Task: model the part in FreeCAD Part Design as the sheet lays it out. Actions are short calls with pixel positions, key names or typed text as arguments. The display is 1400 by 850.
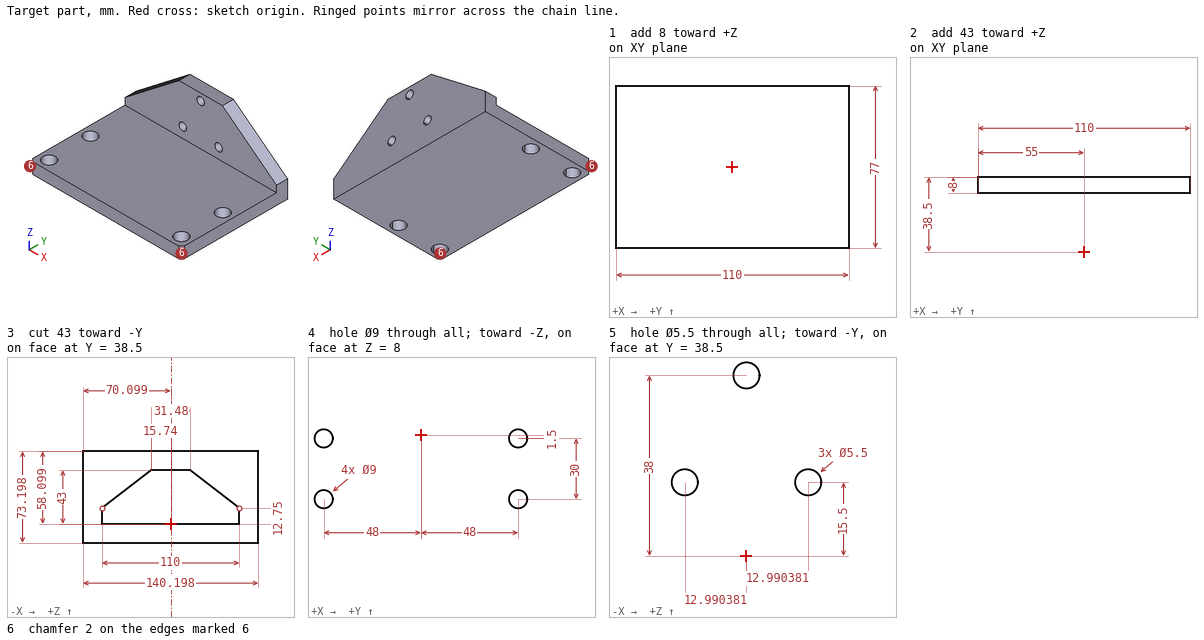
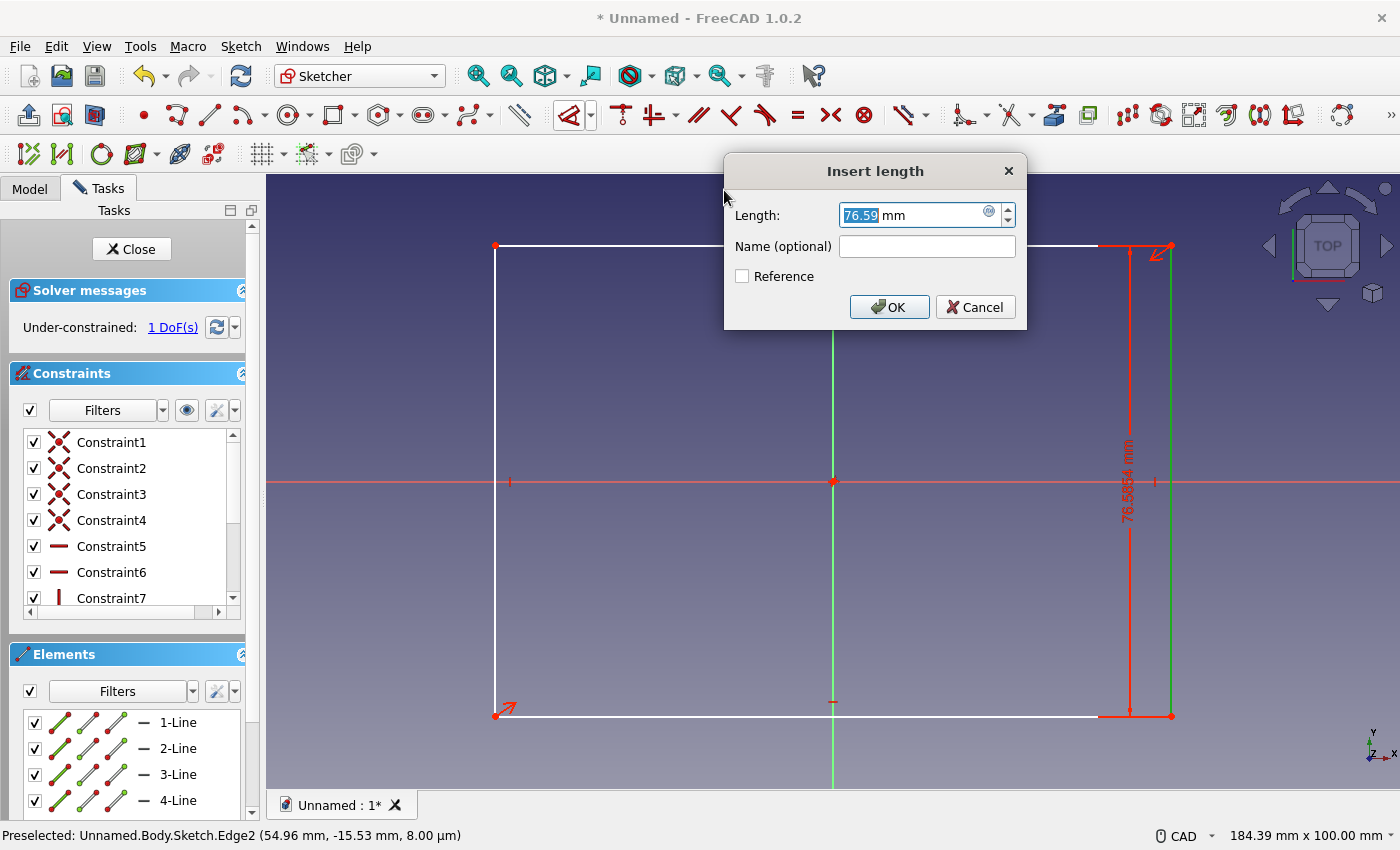
text(77)
key(Return)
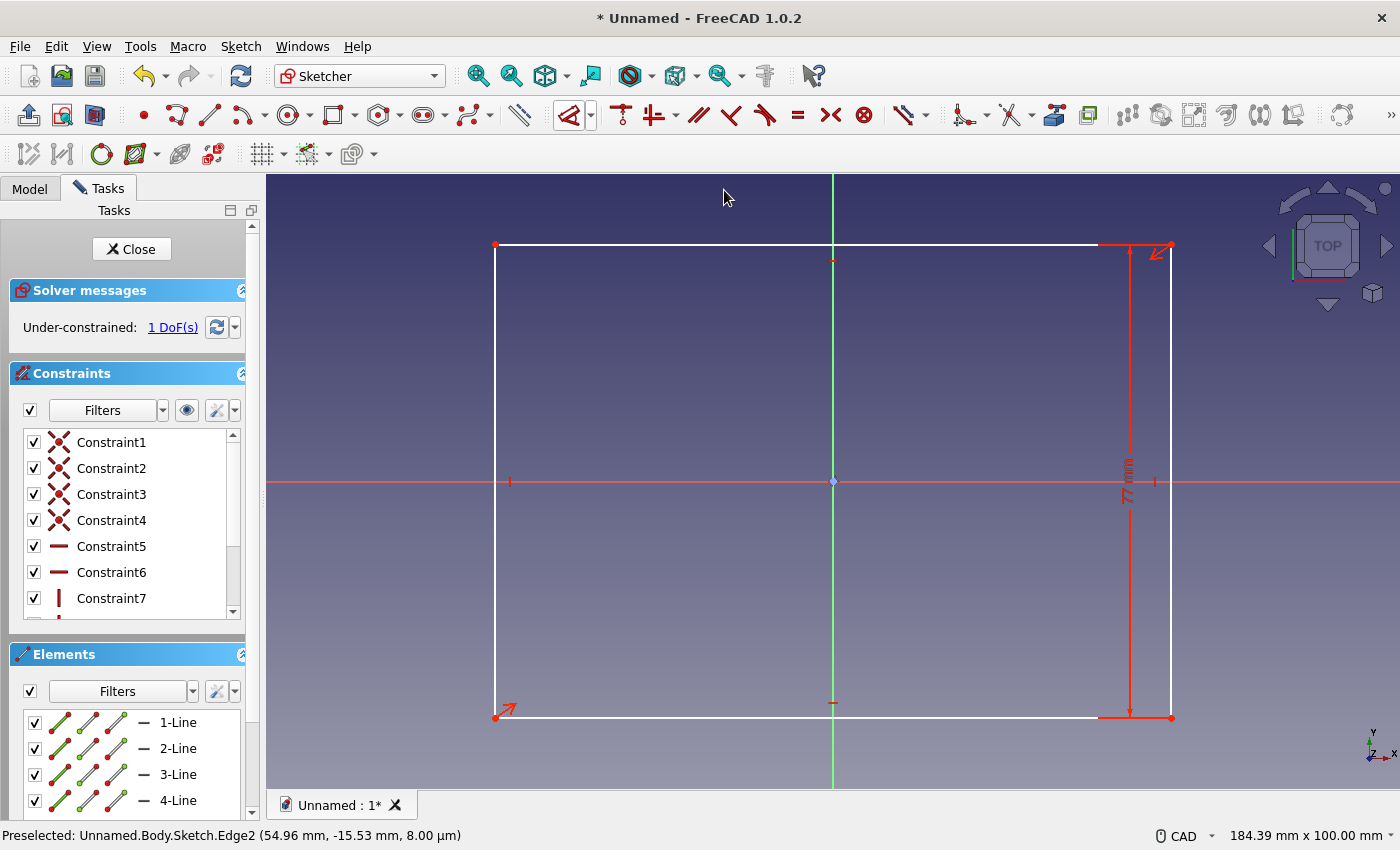
click(698, 718)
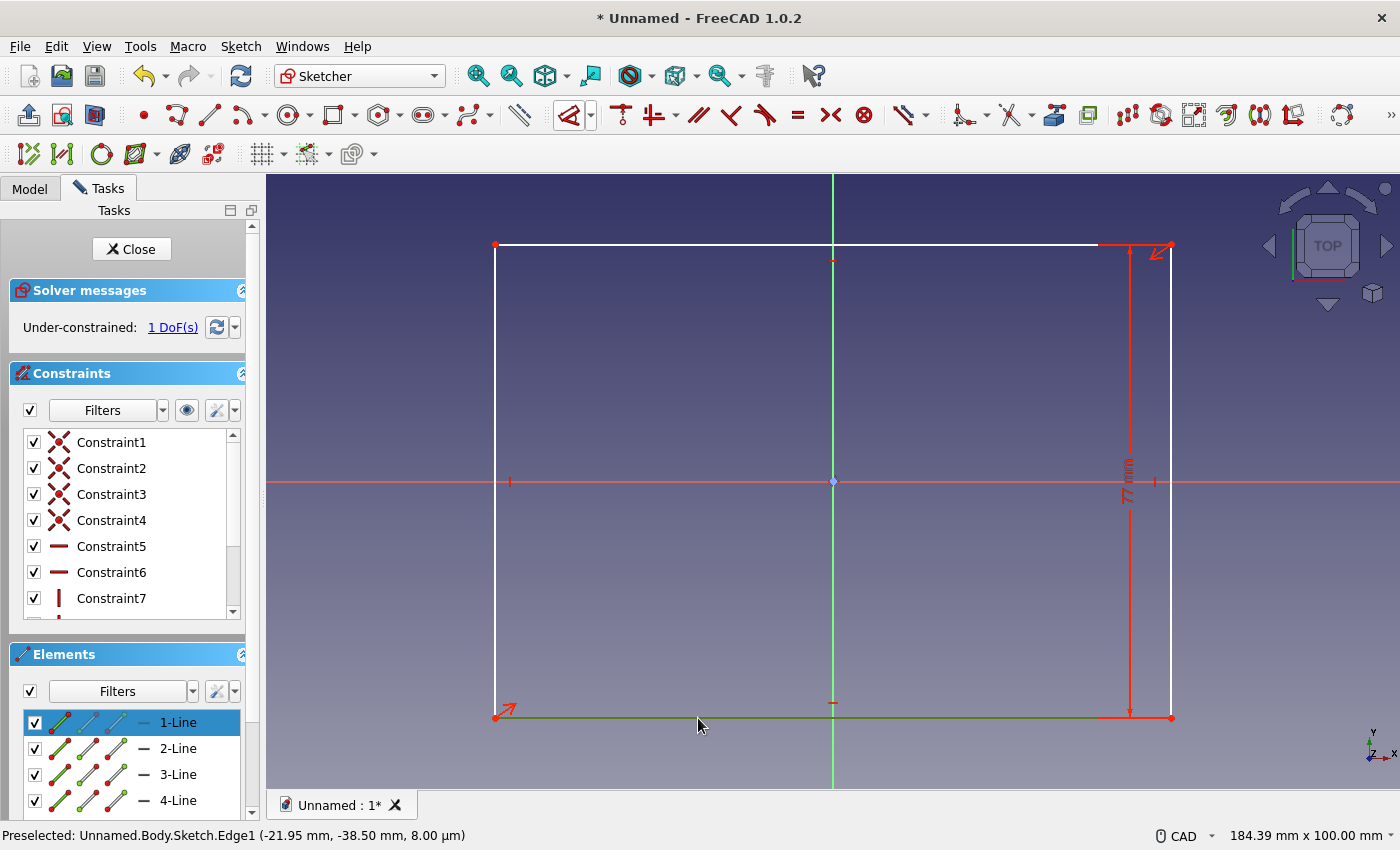
key(l)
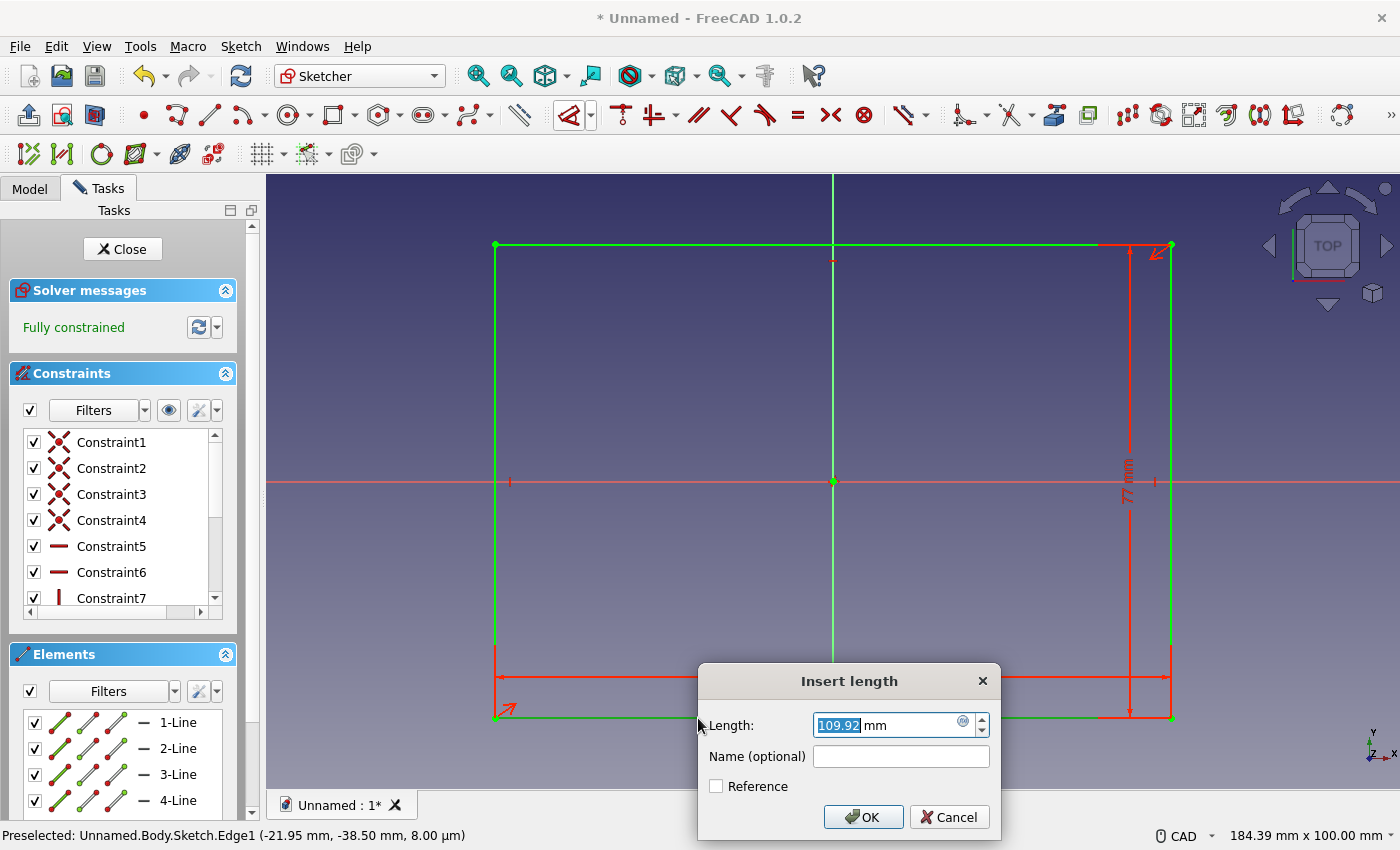
text(110)
key(Return)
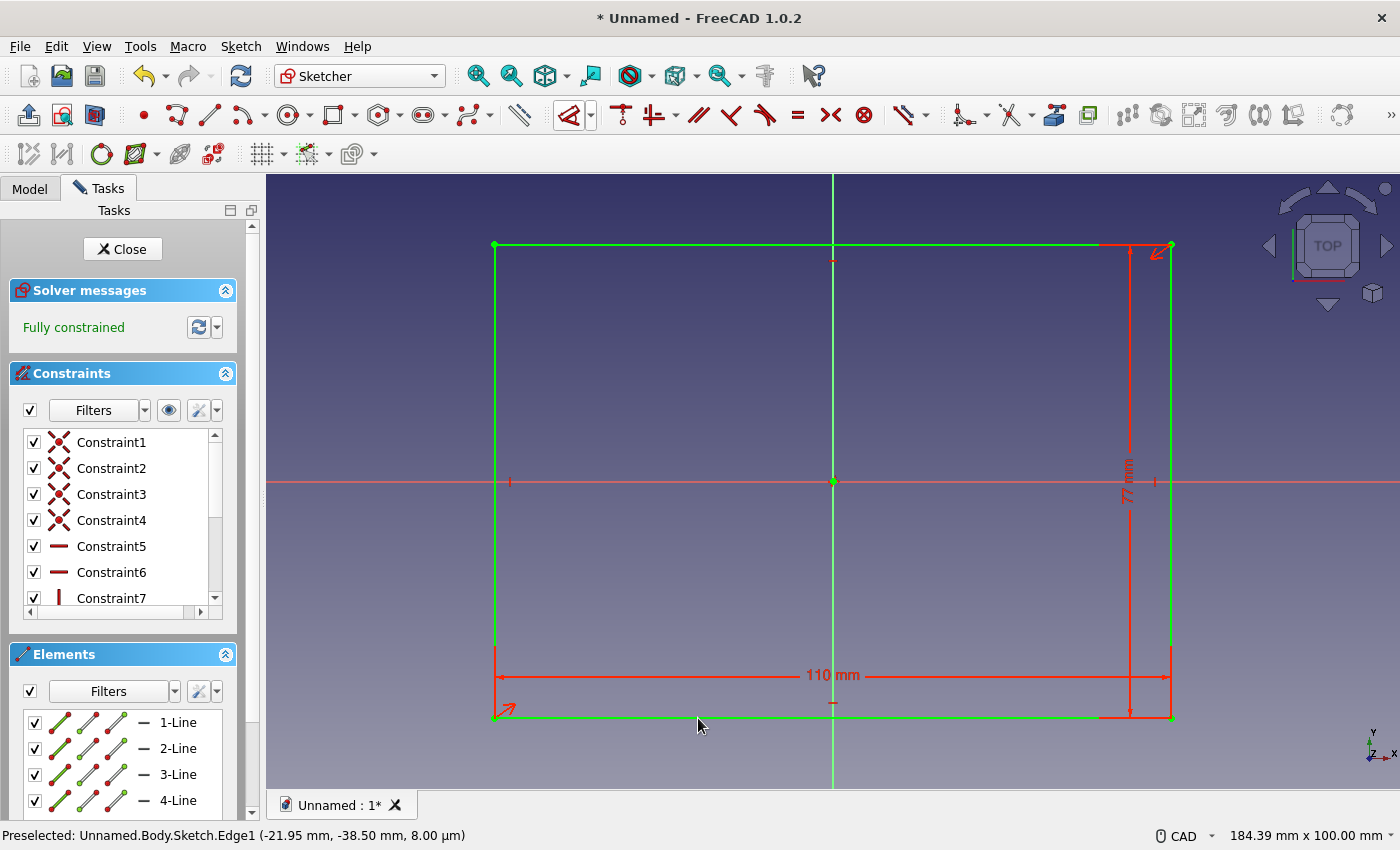
click(123, 249)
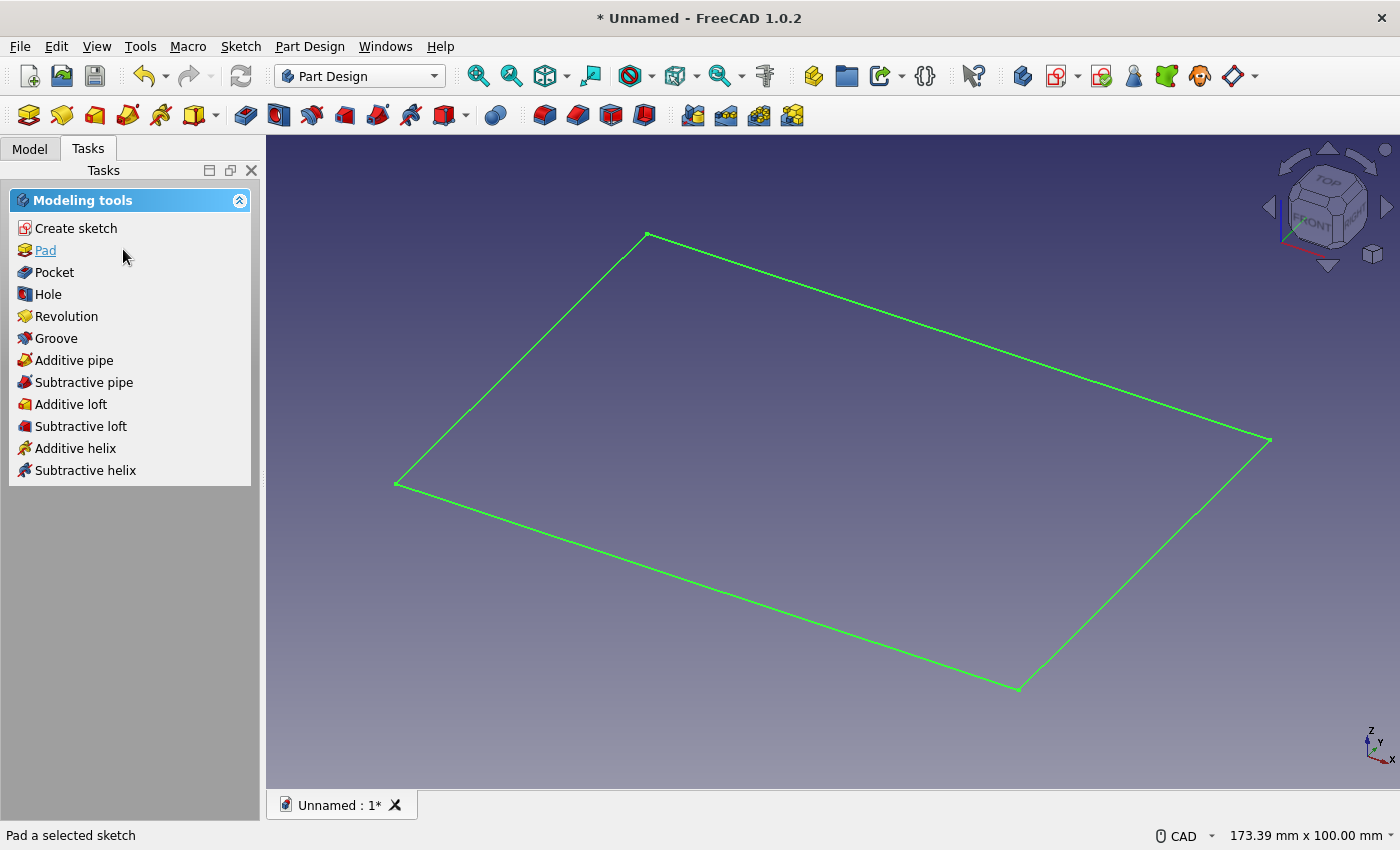
click(29, 116)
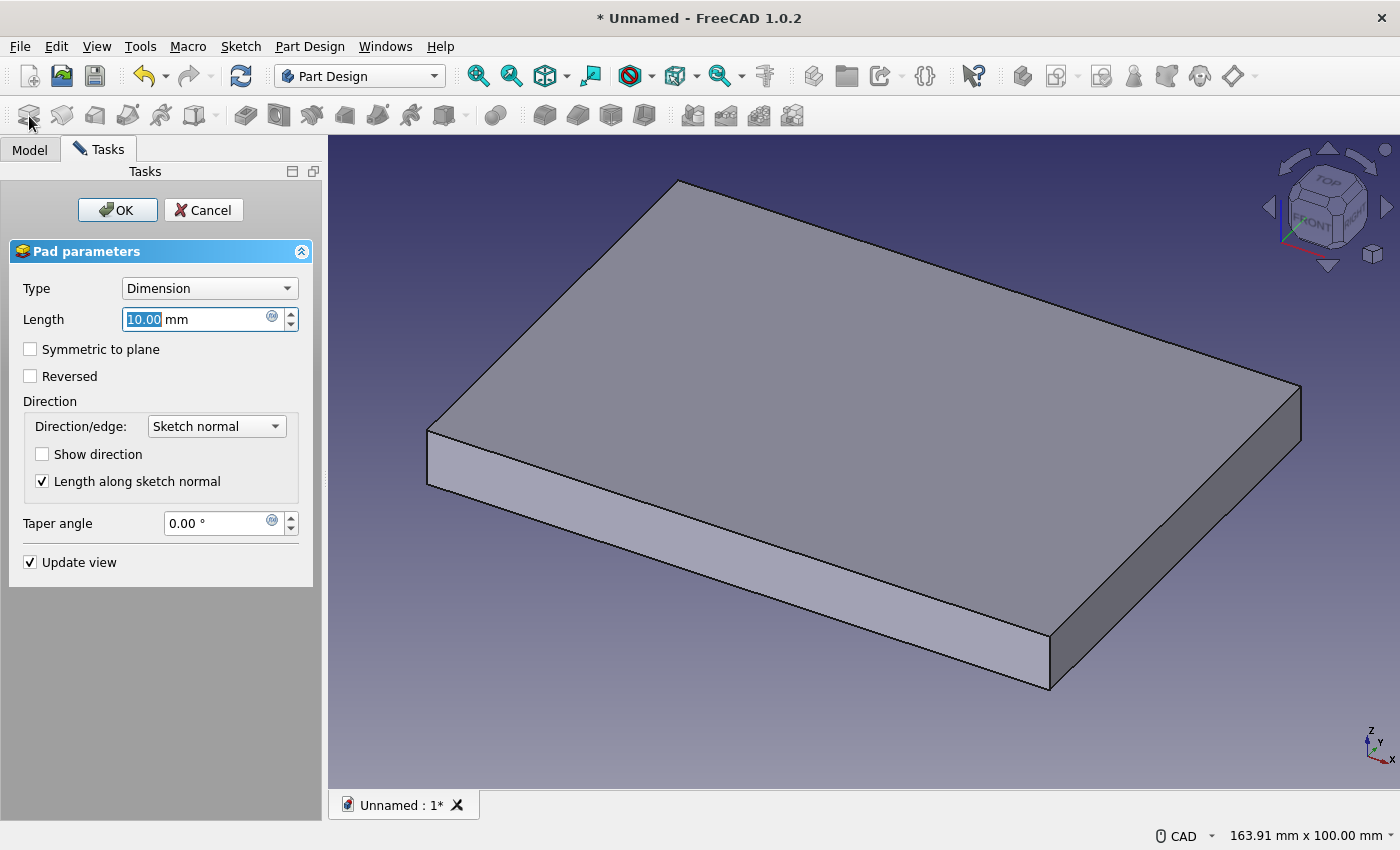
text(8)
key(Tab)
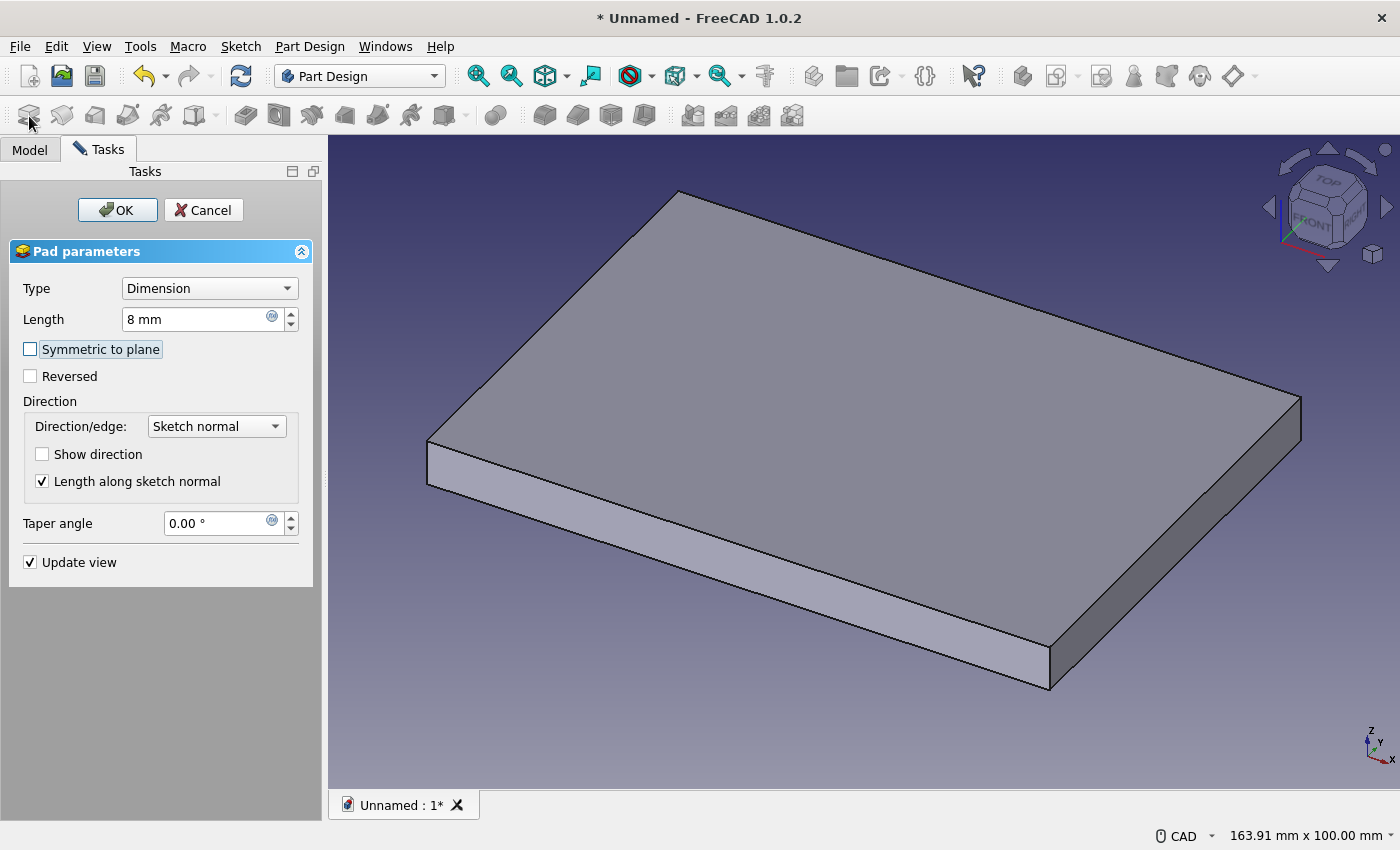
click(118, 210)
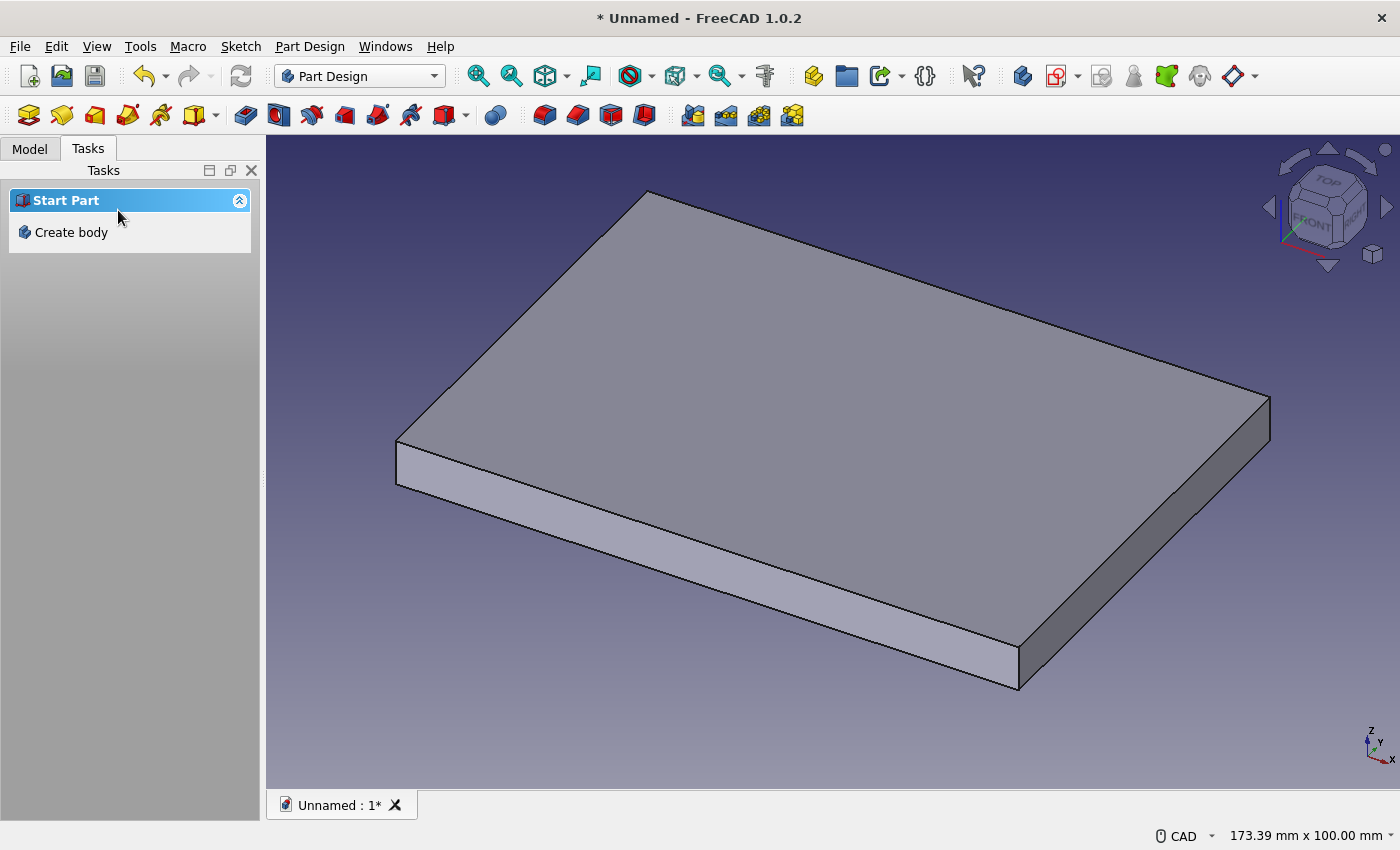
click(1056, 76)